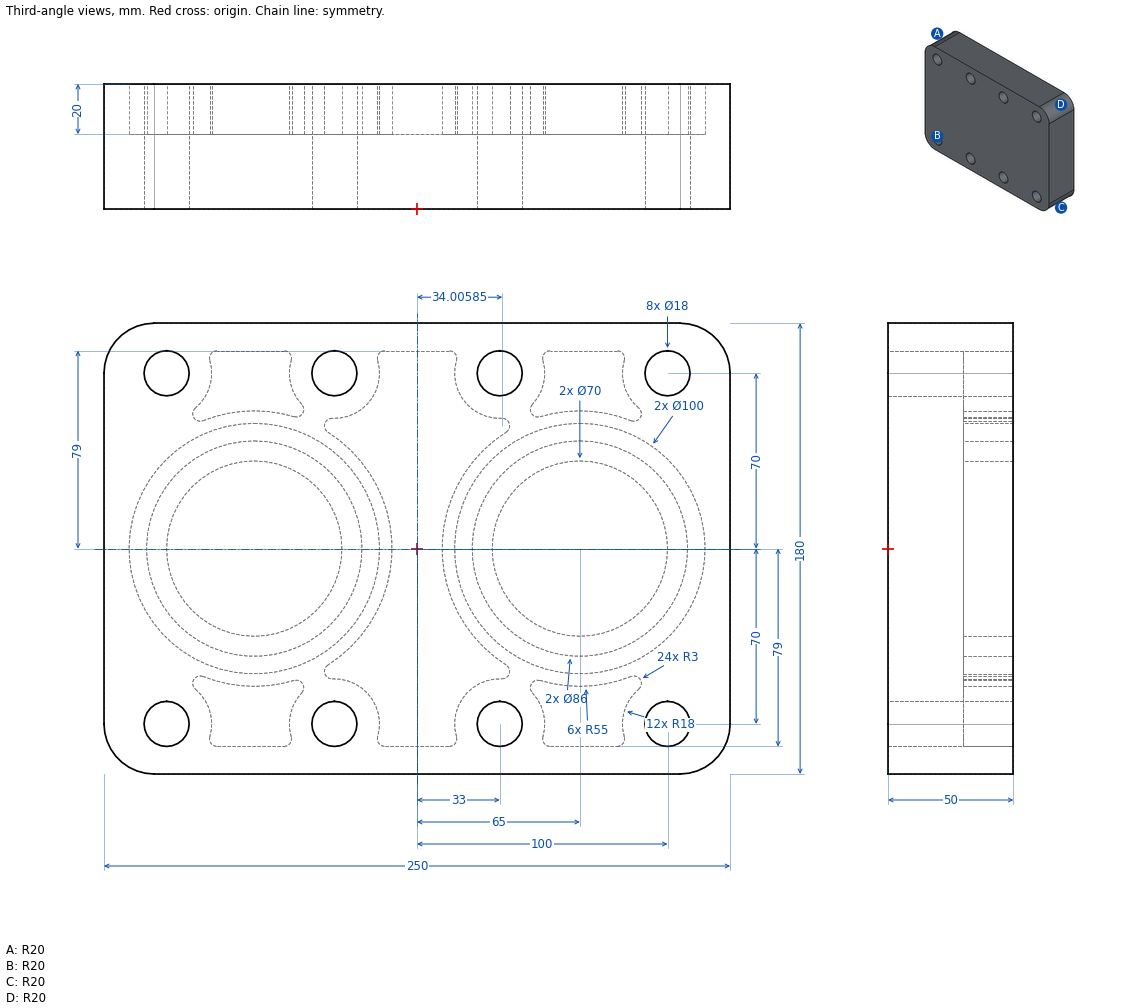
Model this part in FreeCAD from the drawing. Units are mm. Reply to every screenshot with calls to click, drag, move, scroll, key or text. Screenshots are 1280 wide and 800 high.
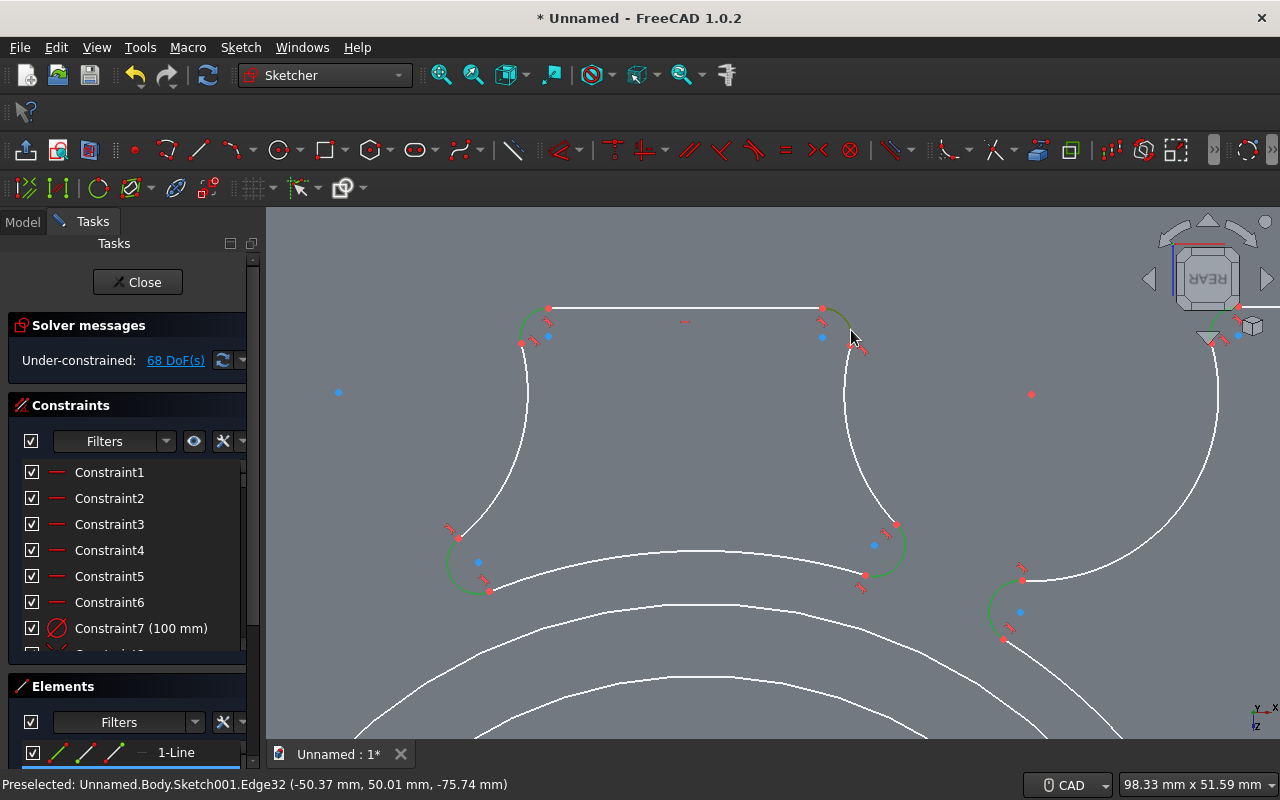
scroll(536, 310, down, 8)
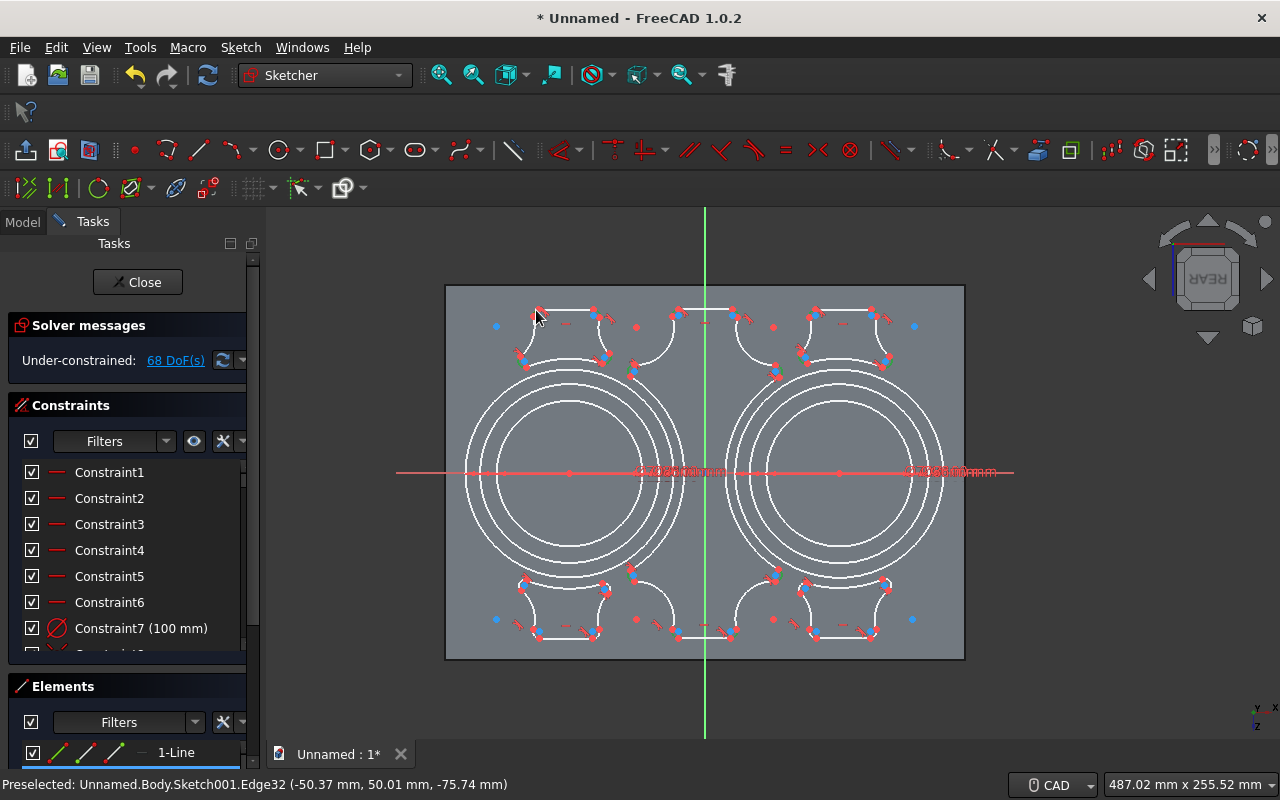
scroll(596, 638, up, 7)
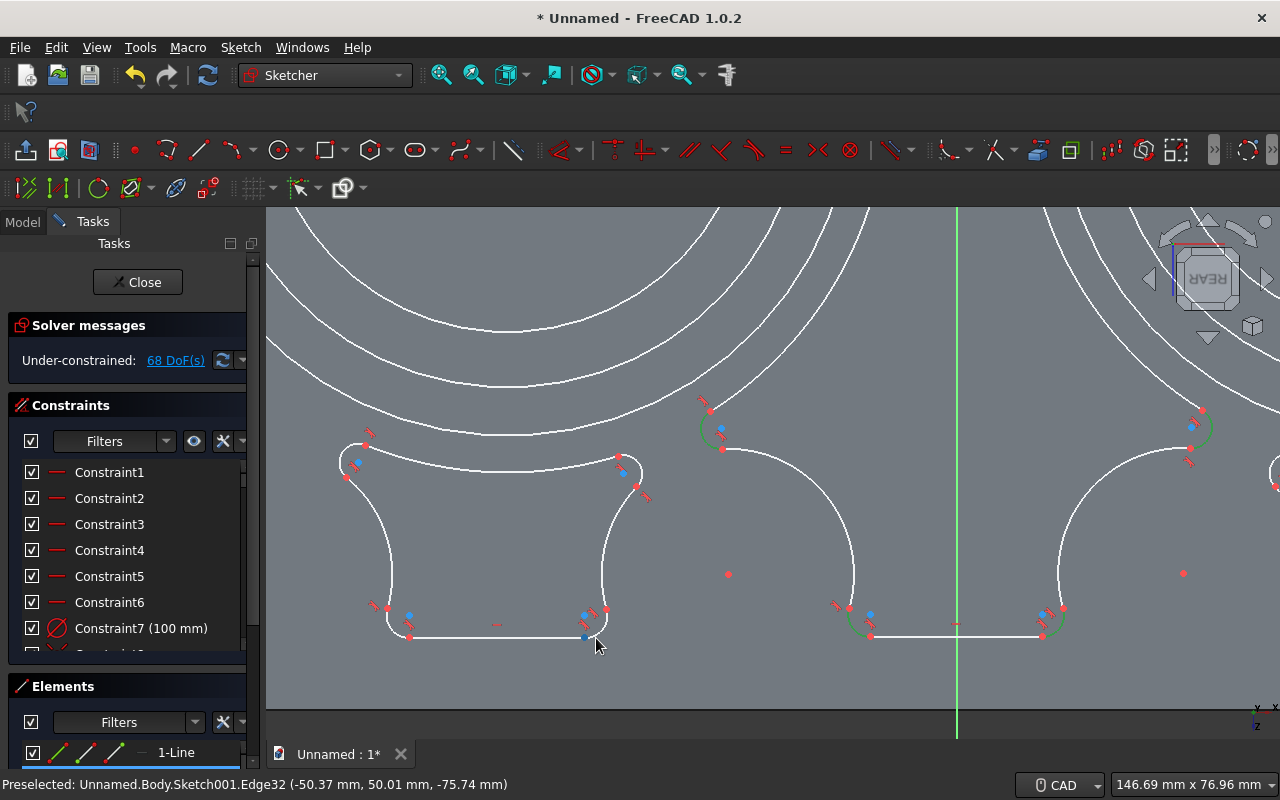
click(597, 634)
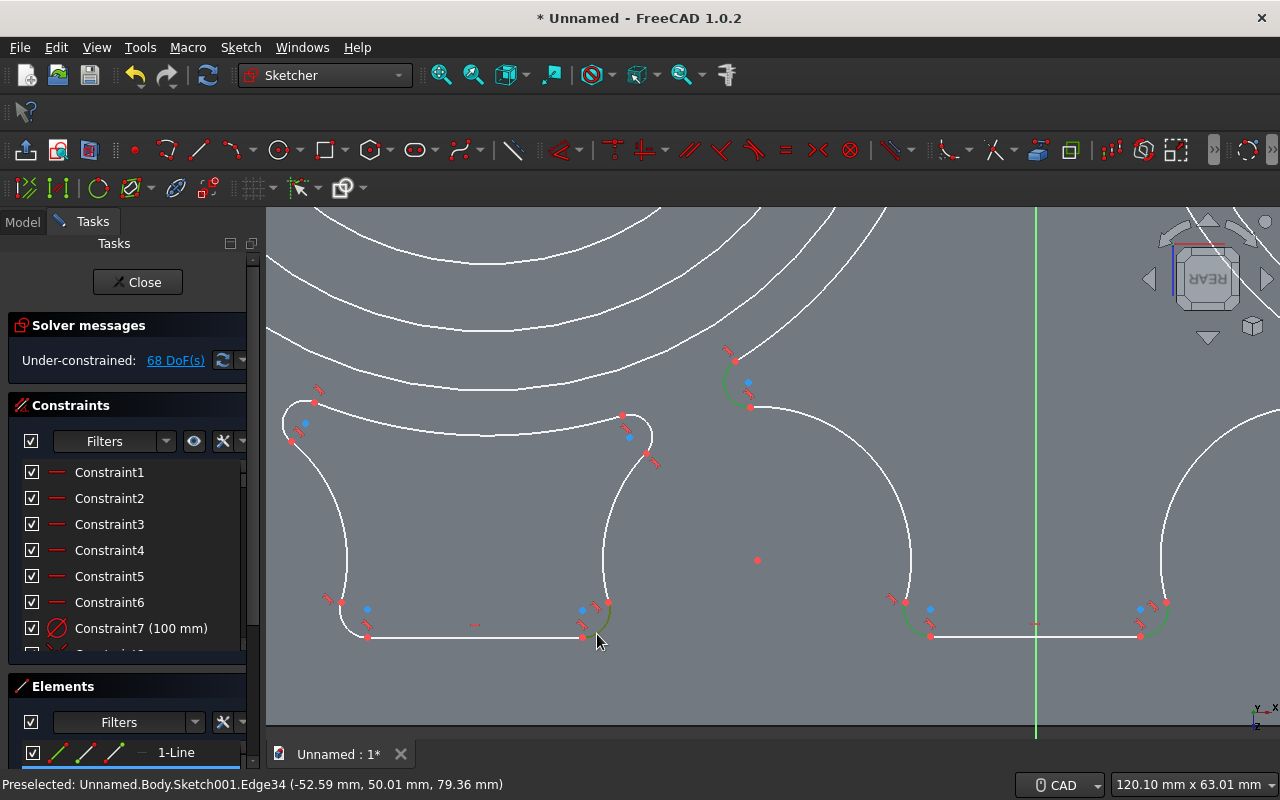
click(652, 437)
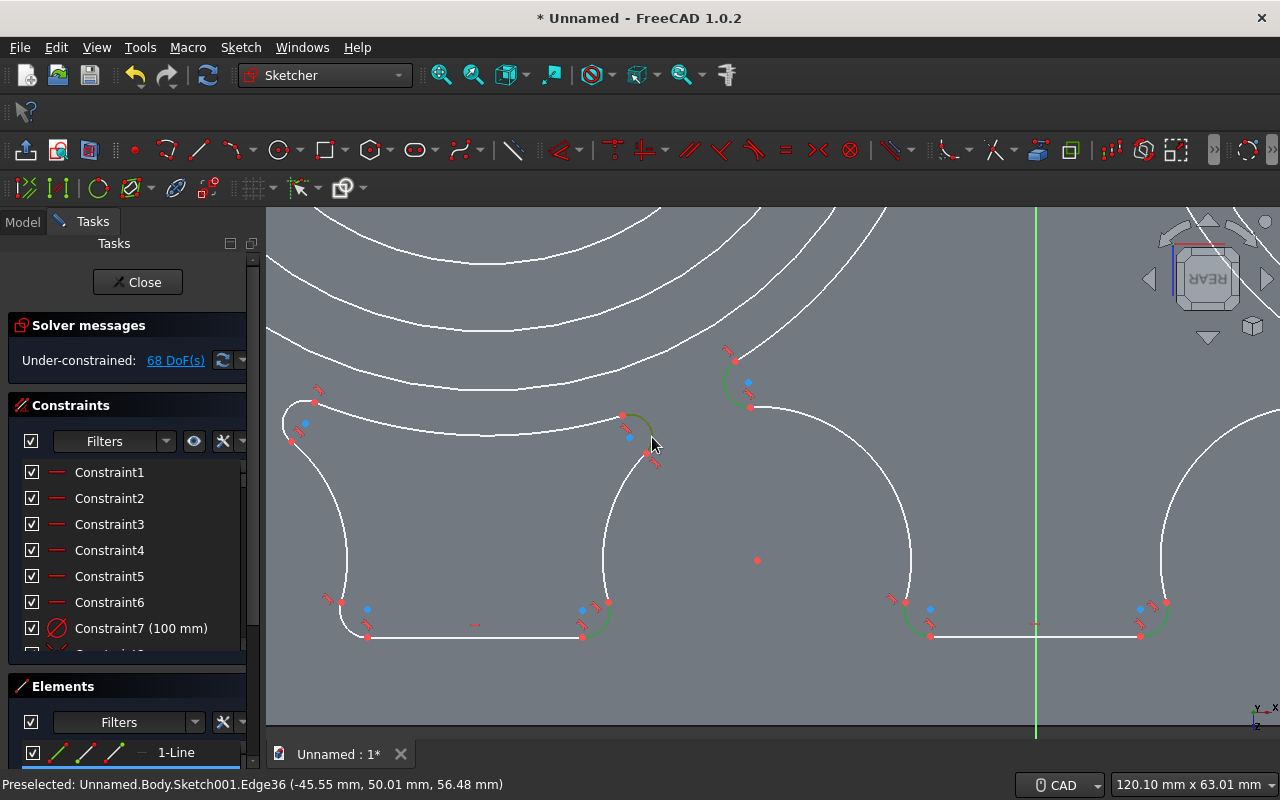
click(295, 403)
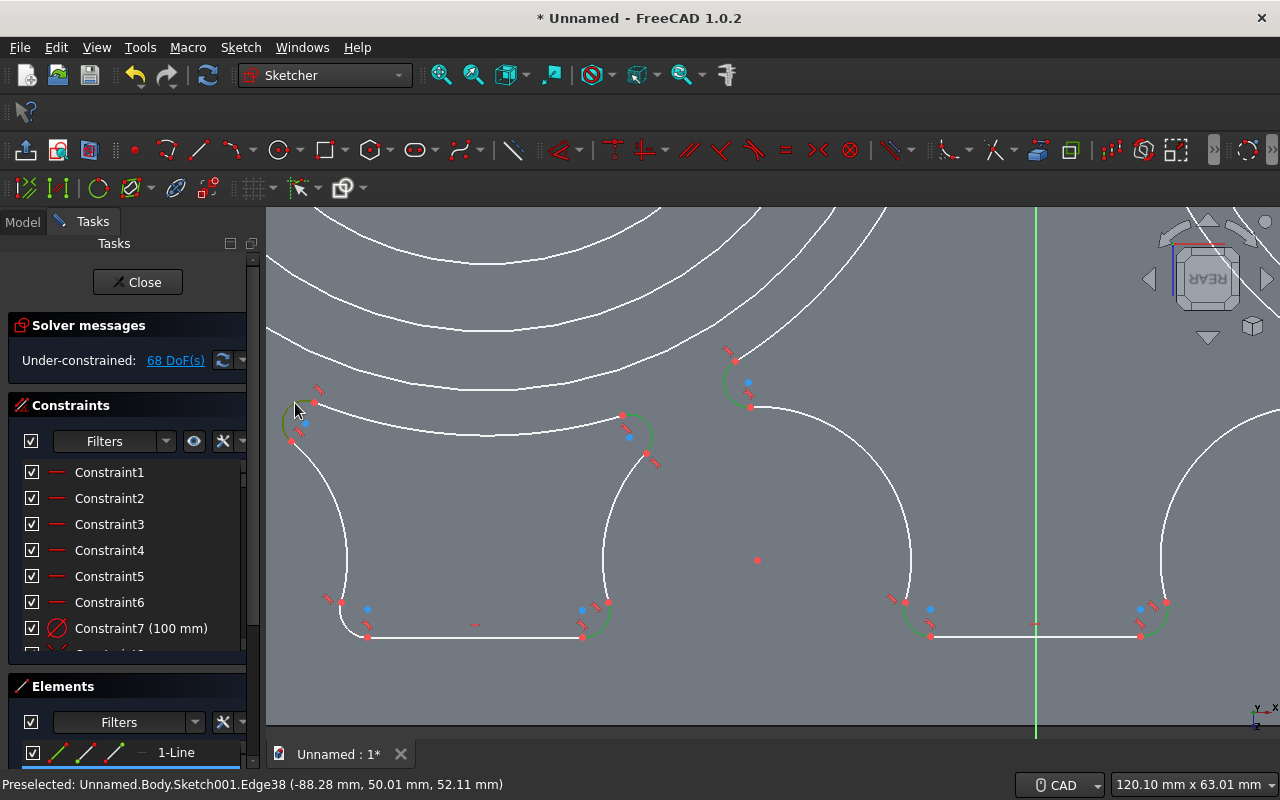
click(341, 618)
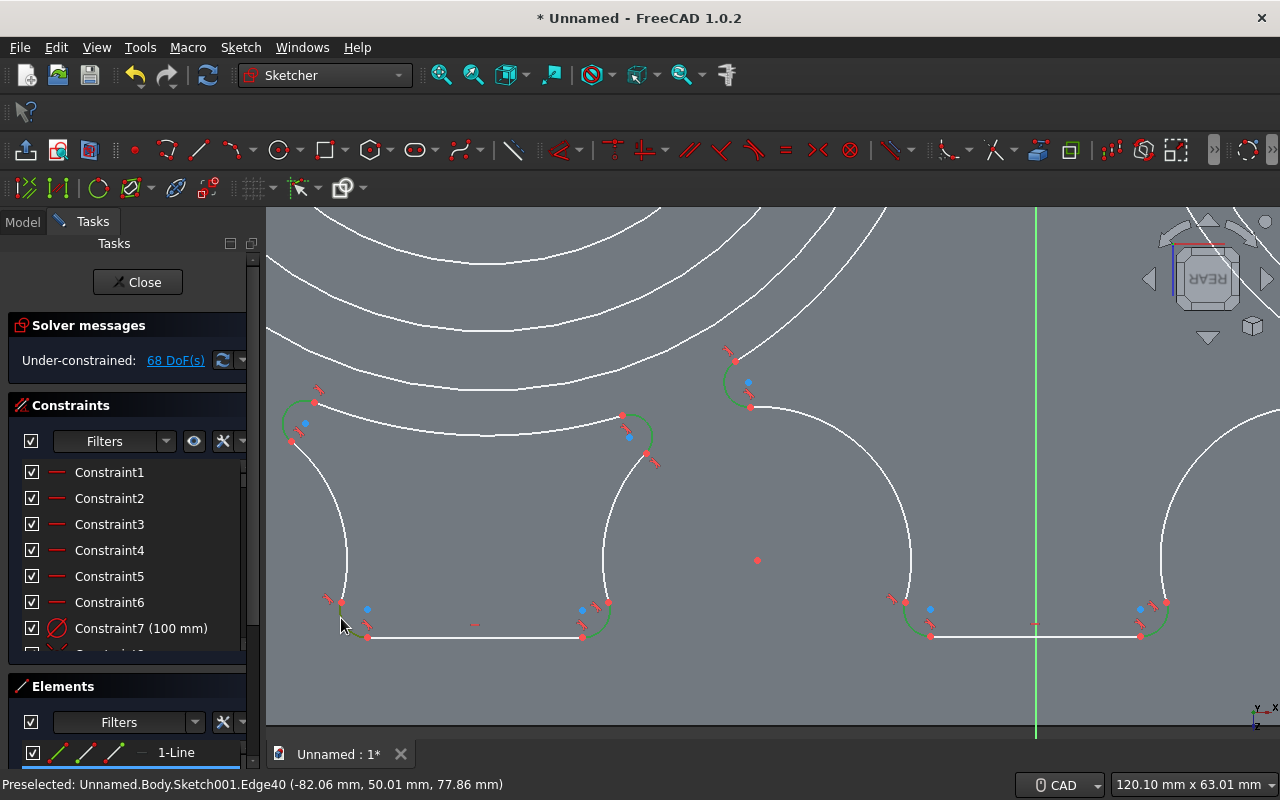
scroll(596, 639, down, 7)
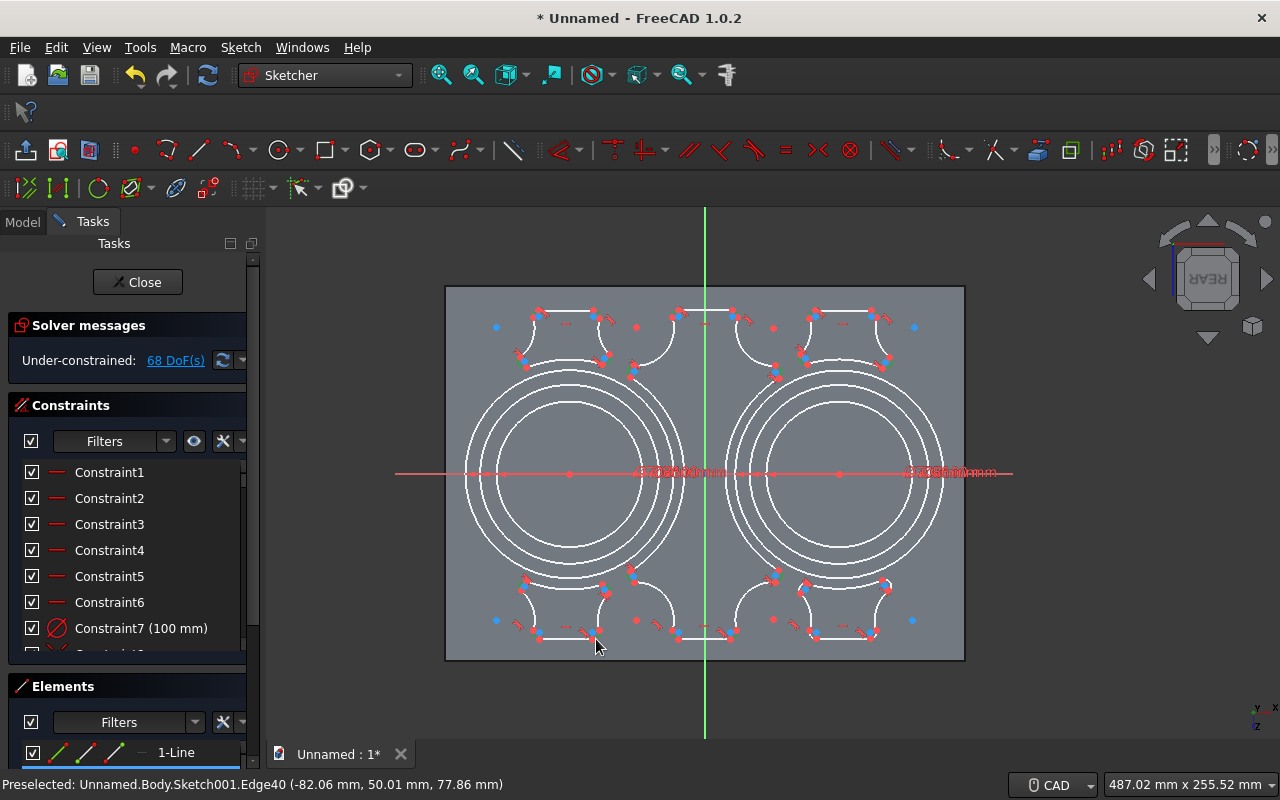
scroll(873, 638, up, 7)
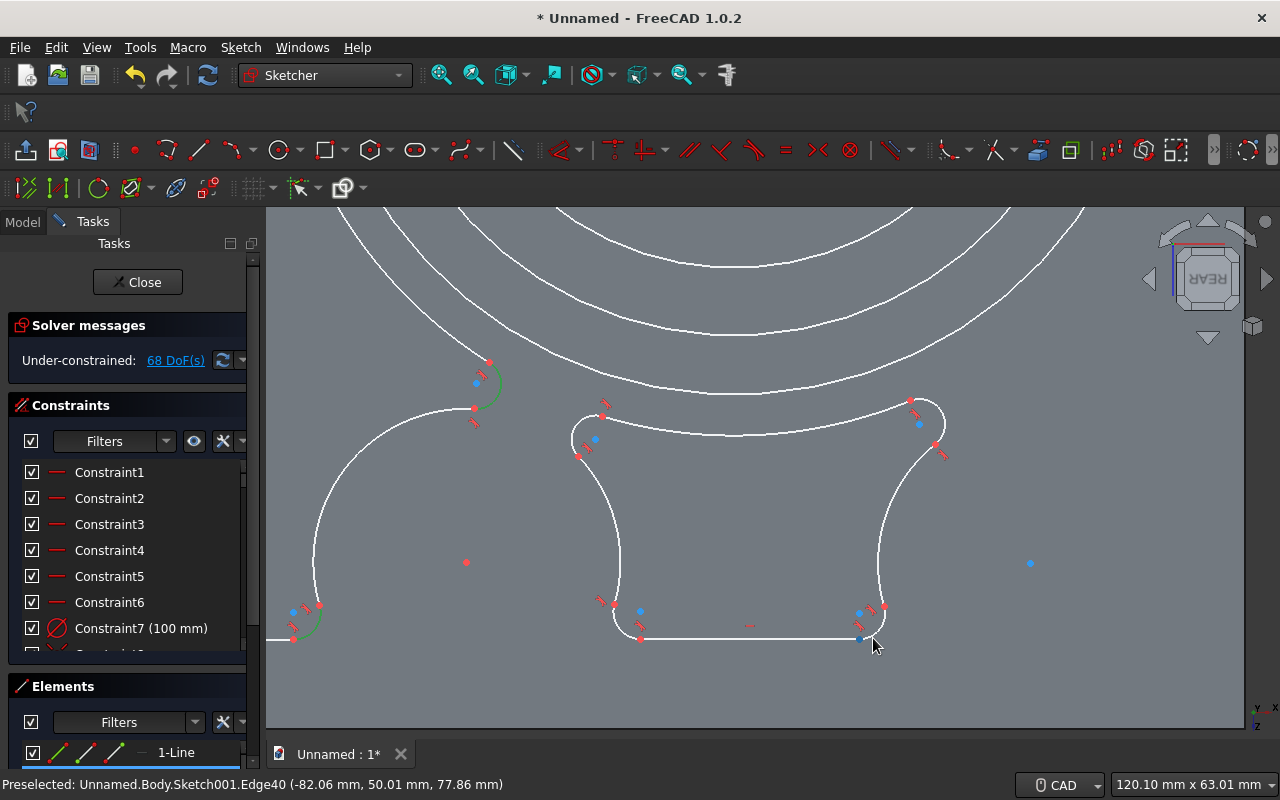
click(873, 635)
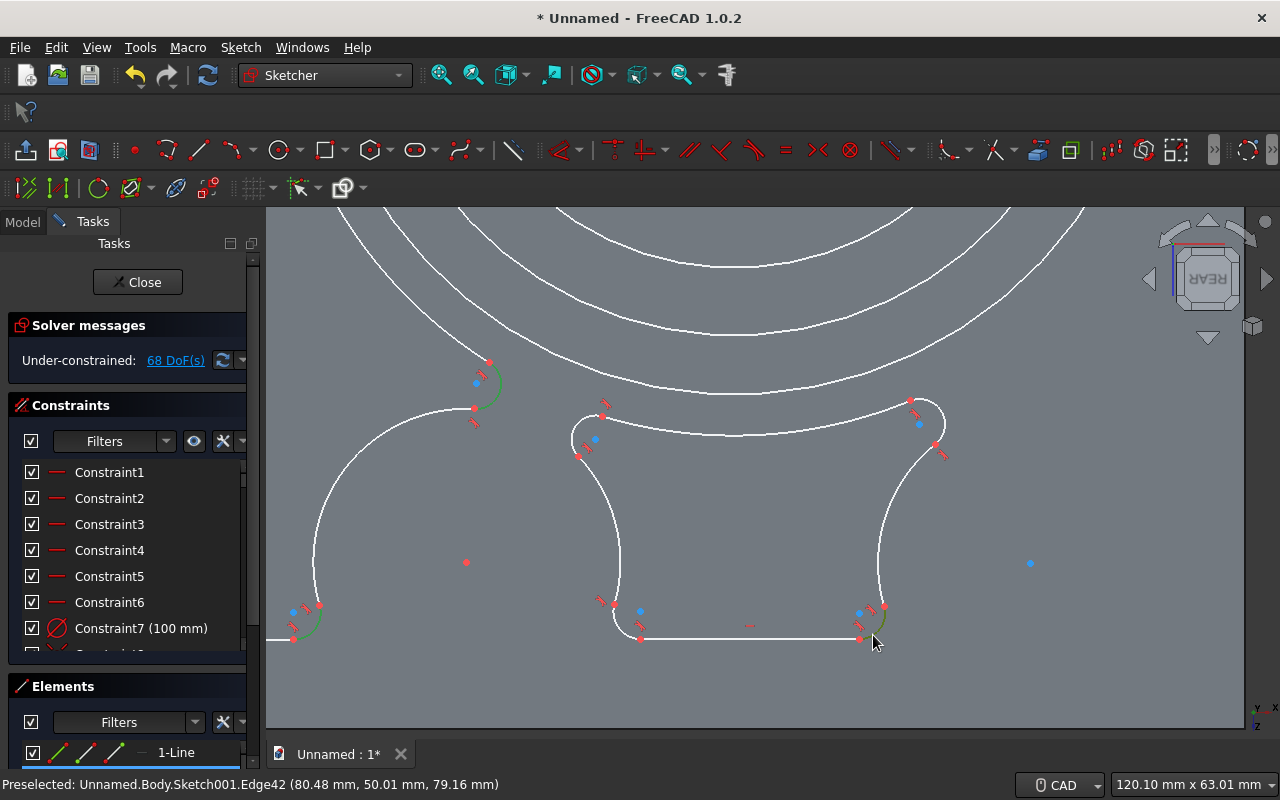
click(945, 425)